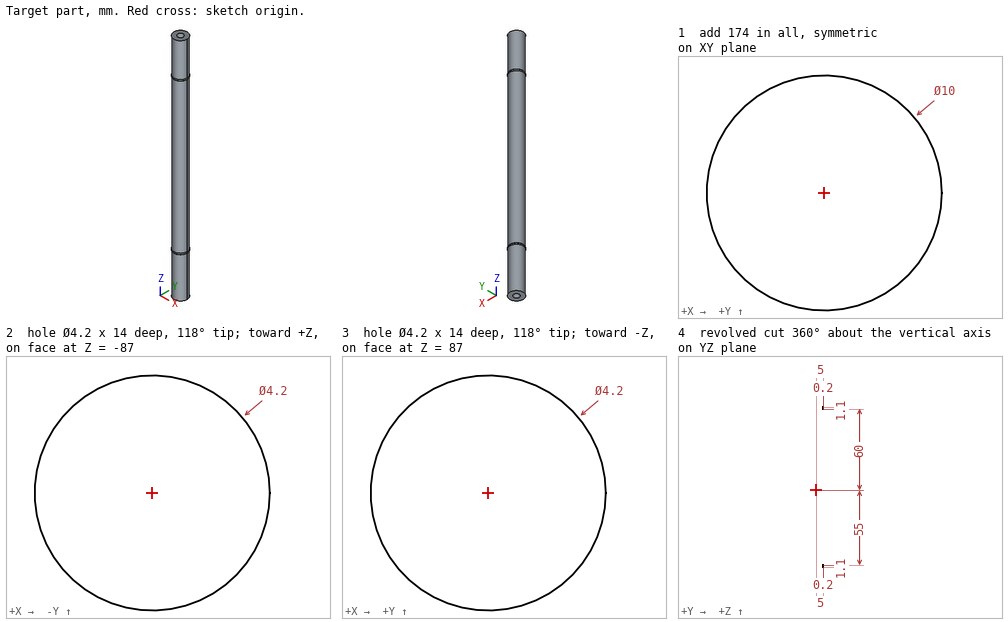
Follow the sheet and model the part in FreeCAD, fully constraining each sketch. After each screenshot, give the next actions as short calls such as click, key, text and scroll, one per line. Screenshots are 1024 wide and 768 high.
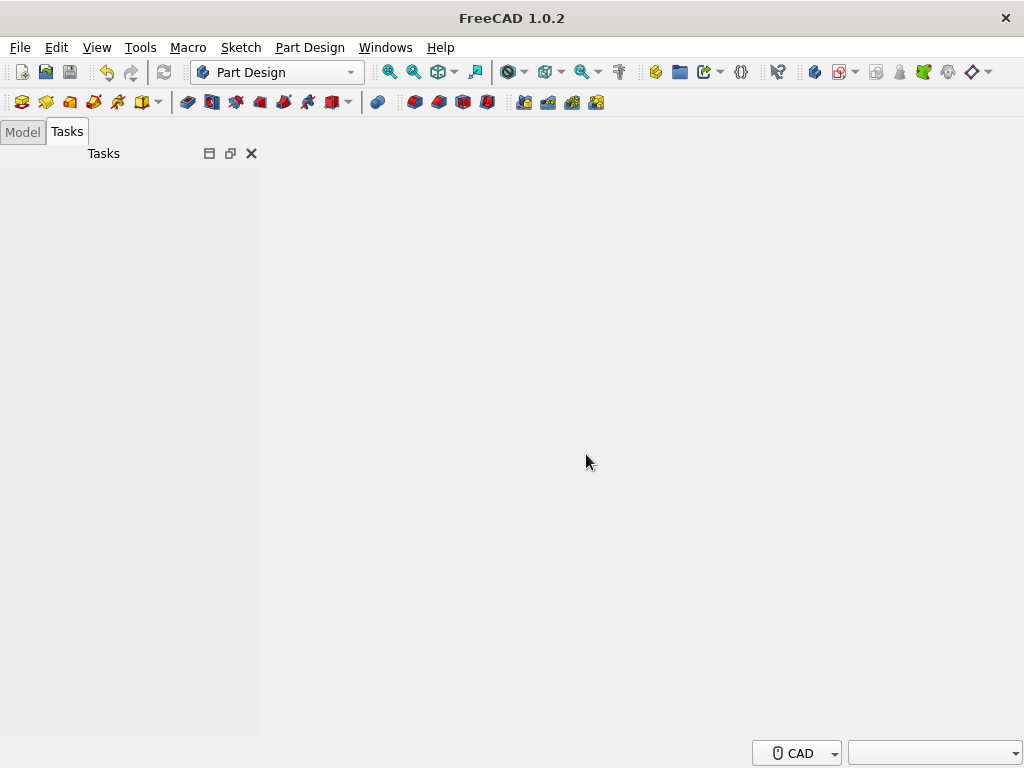
click(22, 72)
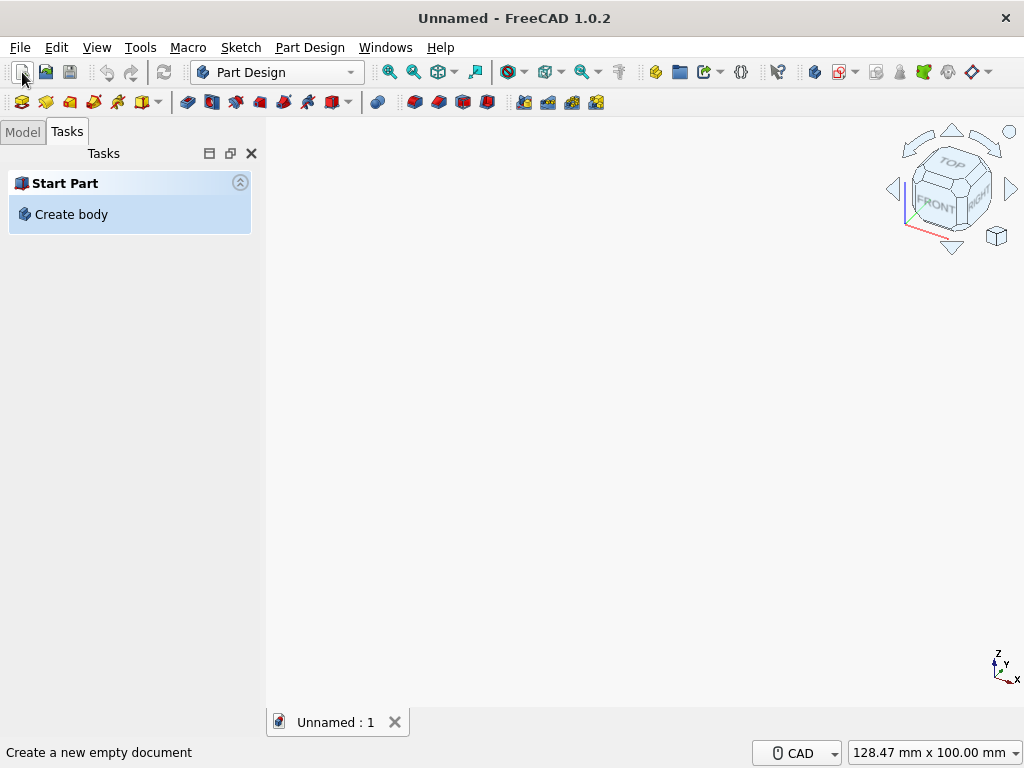
click(840, 72)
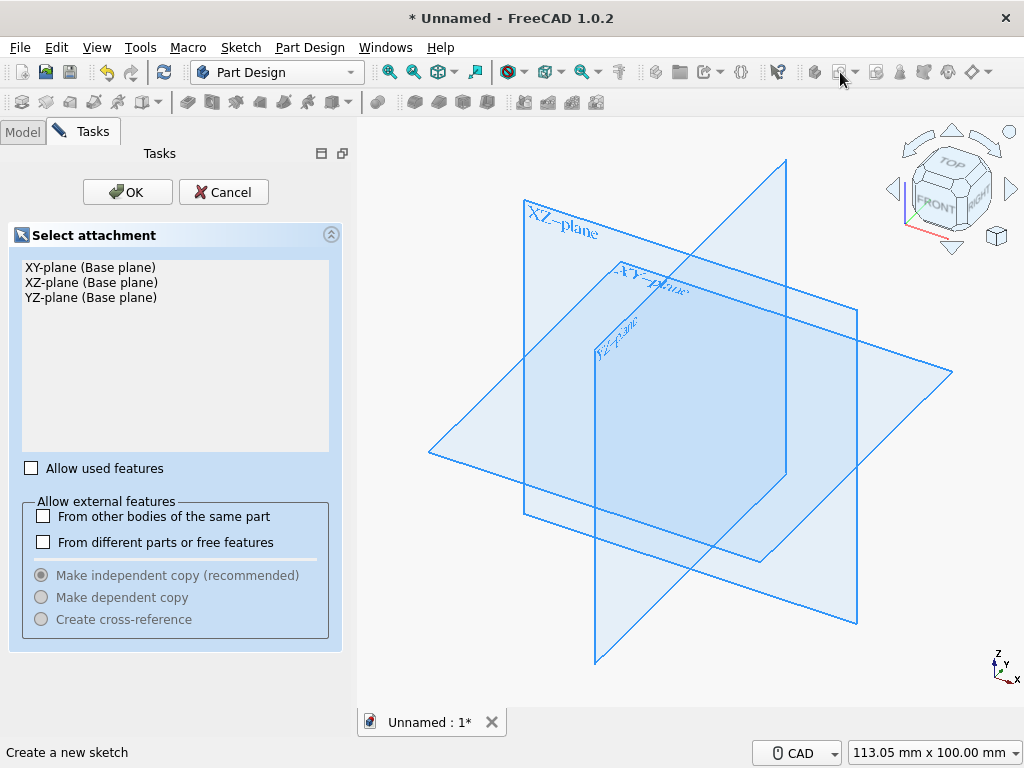
click(82, 268)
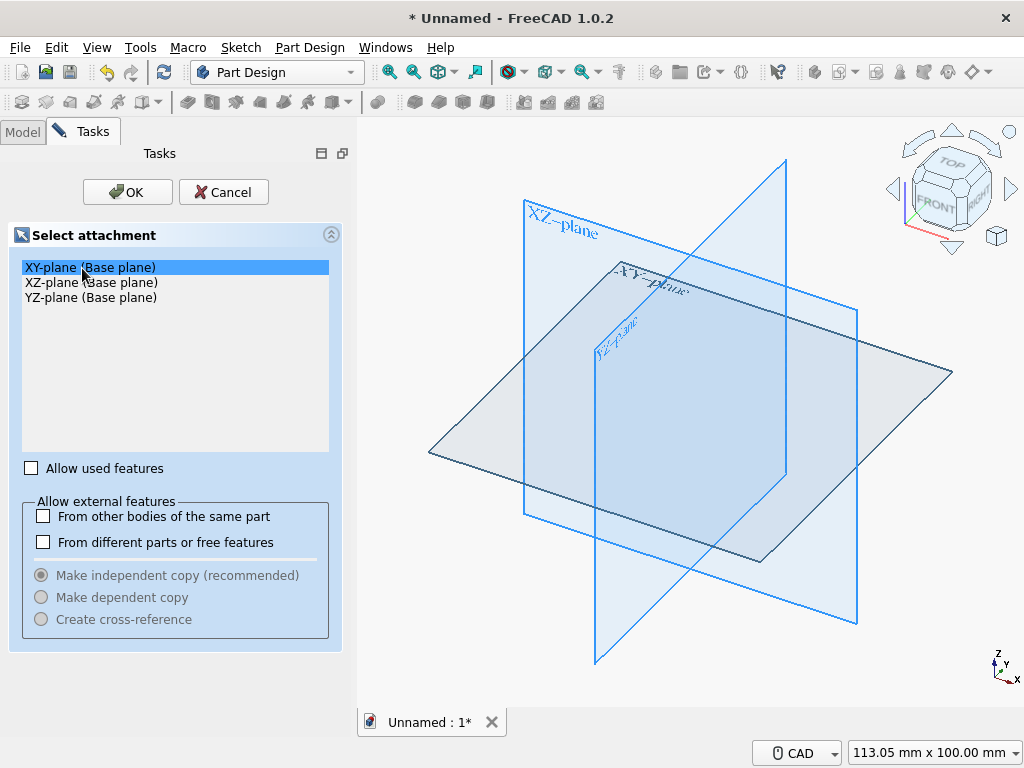
click(128, 192)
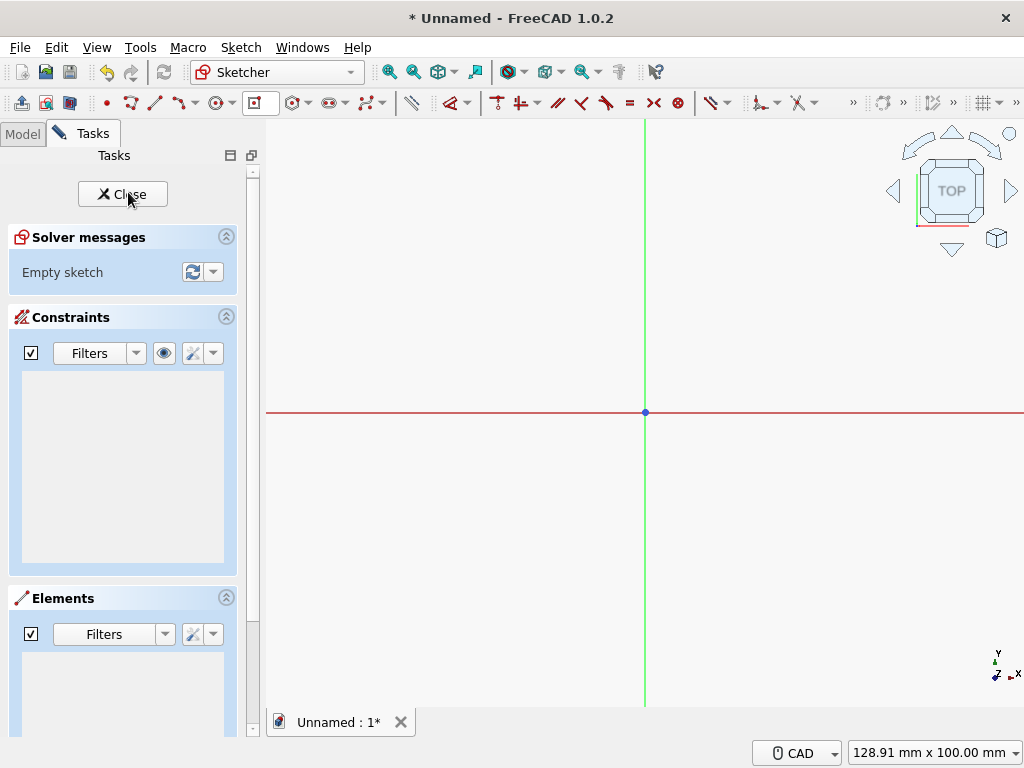
scroll(659, 413, up, 9)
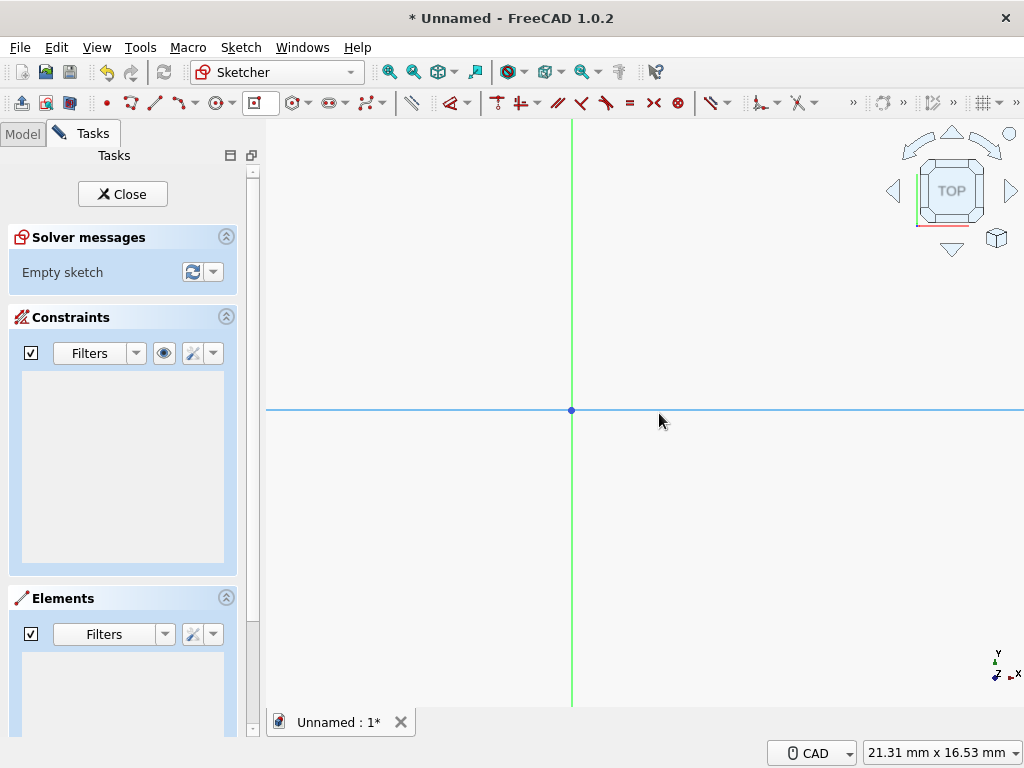
click(216, 104)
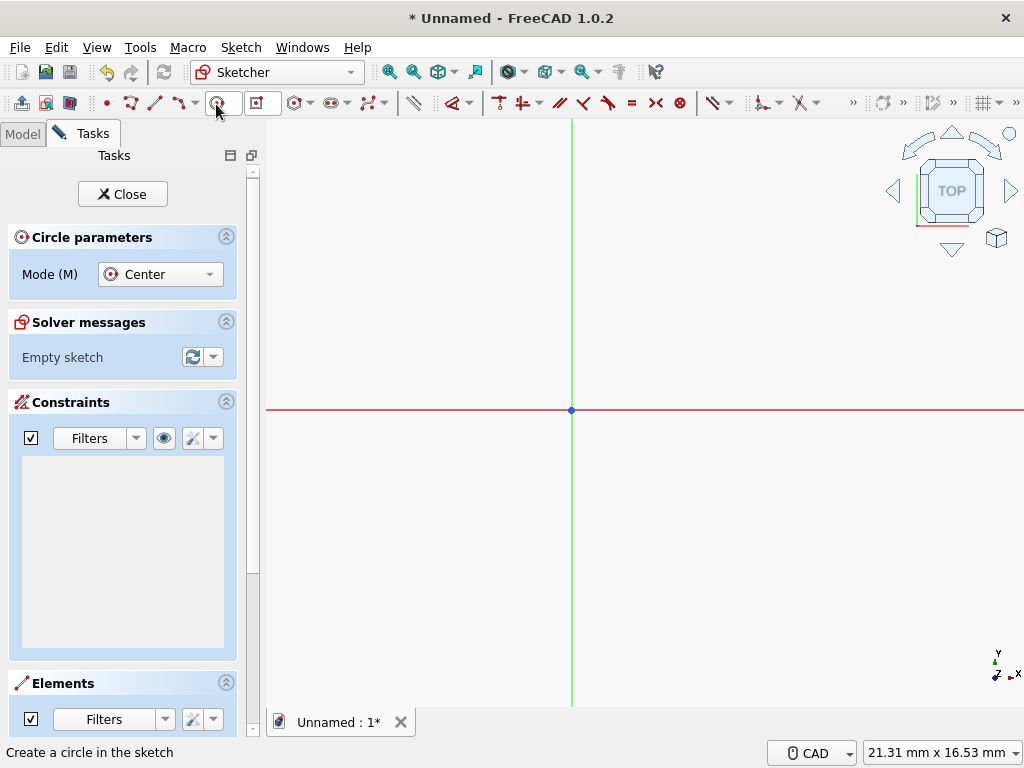
click(572, 410)
move(697, 285)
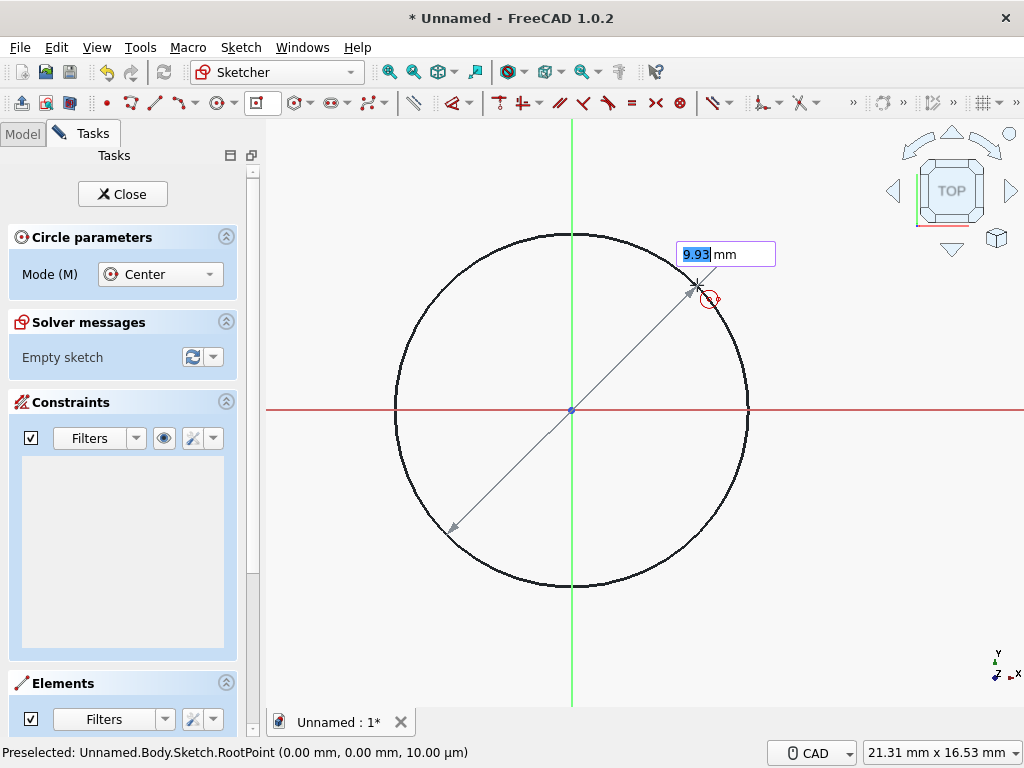
text(10)
key(Return)
key(Escape)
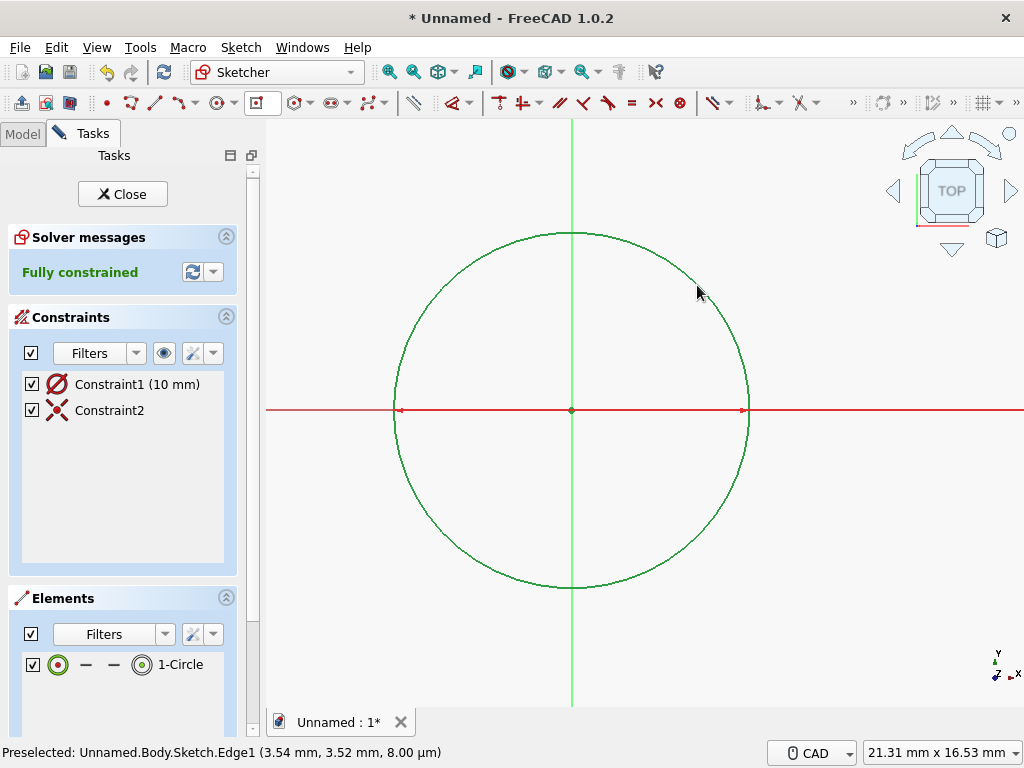
click(123, 194)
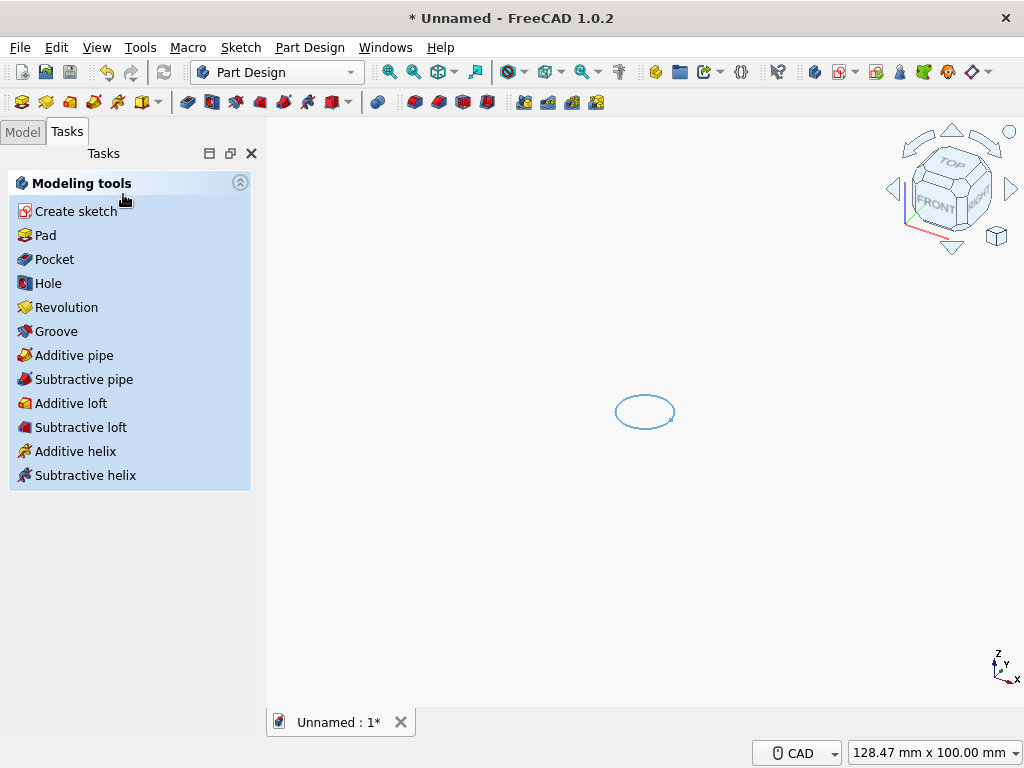
click(22, 102)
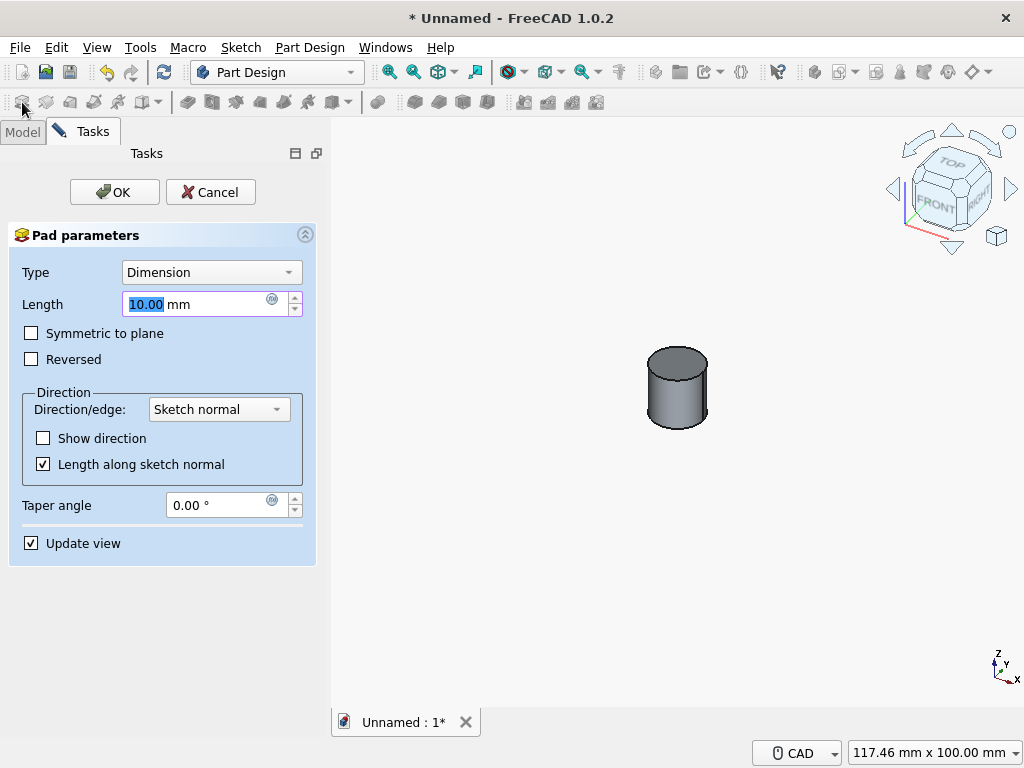
text(174)
key(Tab)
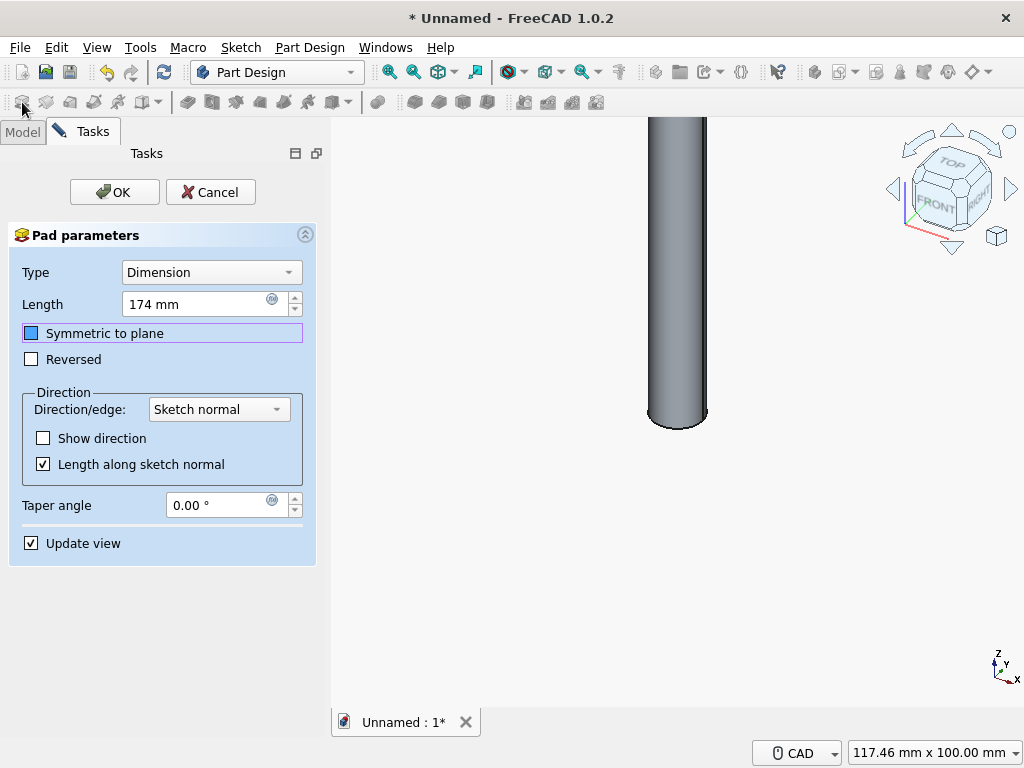
click(30, 333)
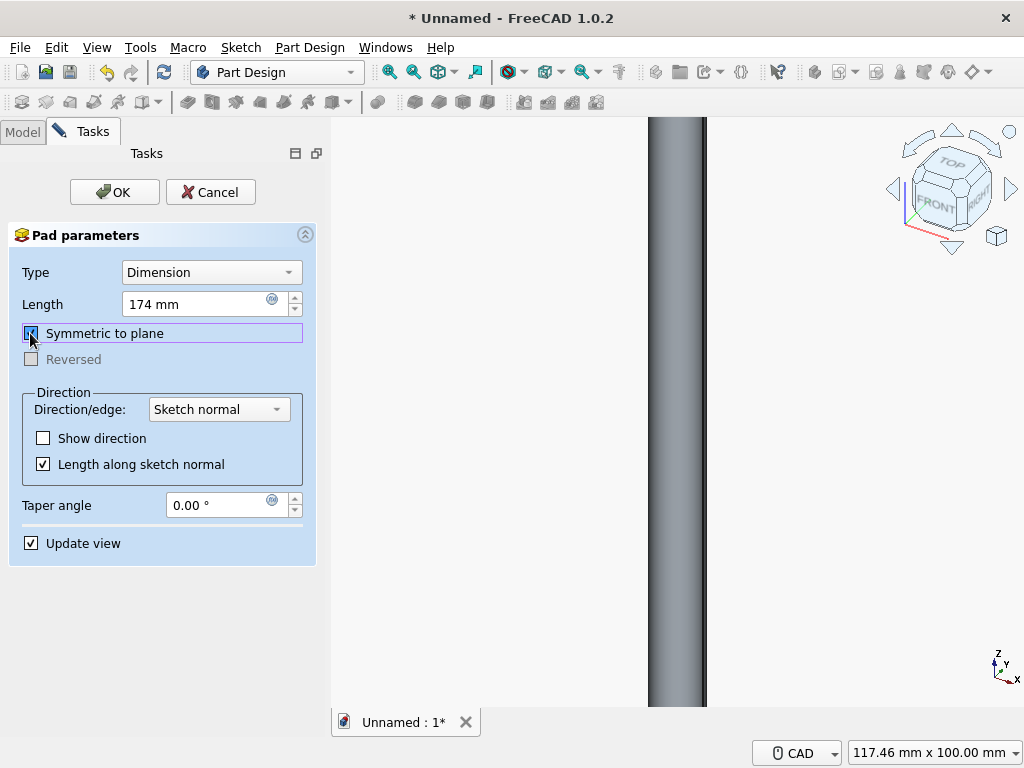
click(115, 192)